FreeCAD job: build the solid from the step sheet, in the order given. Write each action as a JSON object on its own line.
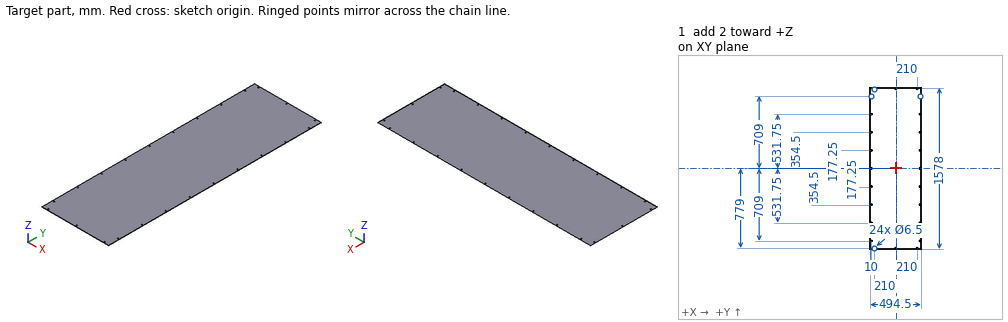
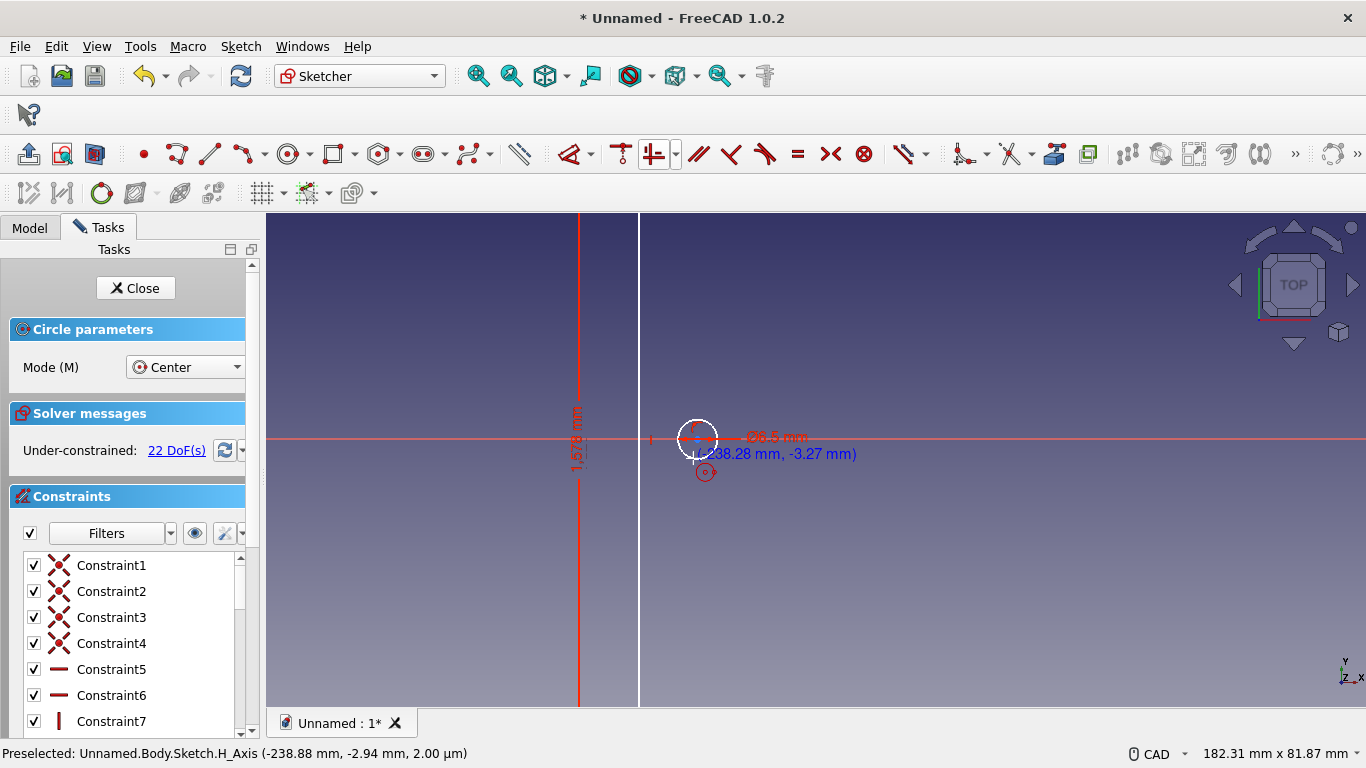
{"action": "scroll", "coordinate": [700, 461], "scroll_direction": "down", "scroll_amount": 17}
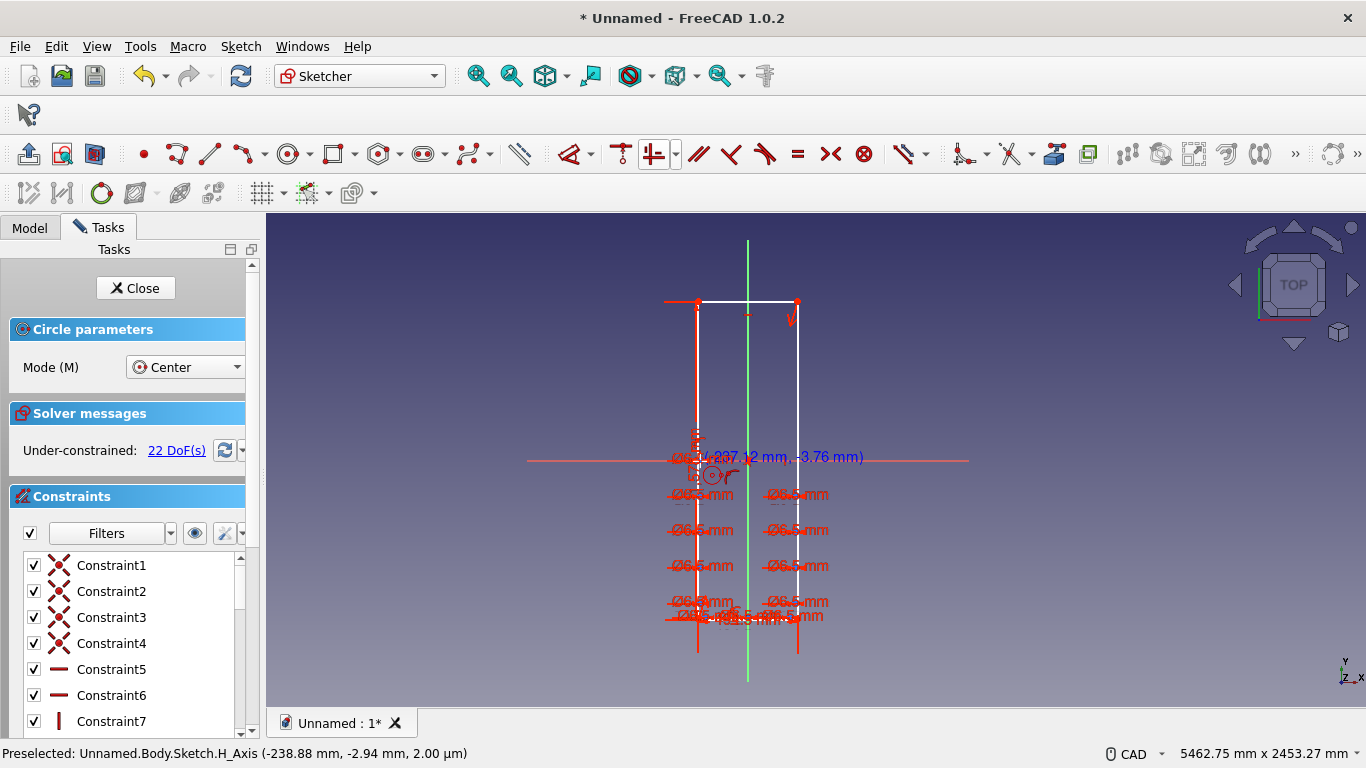
{"action": "scroll", "coordinate": [700, 425], "scroll_direction": "up", "scroll_amount": 18}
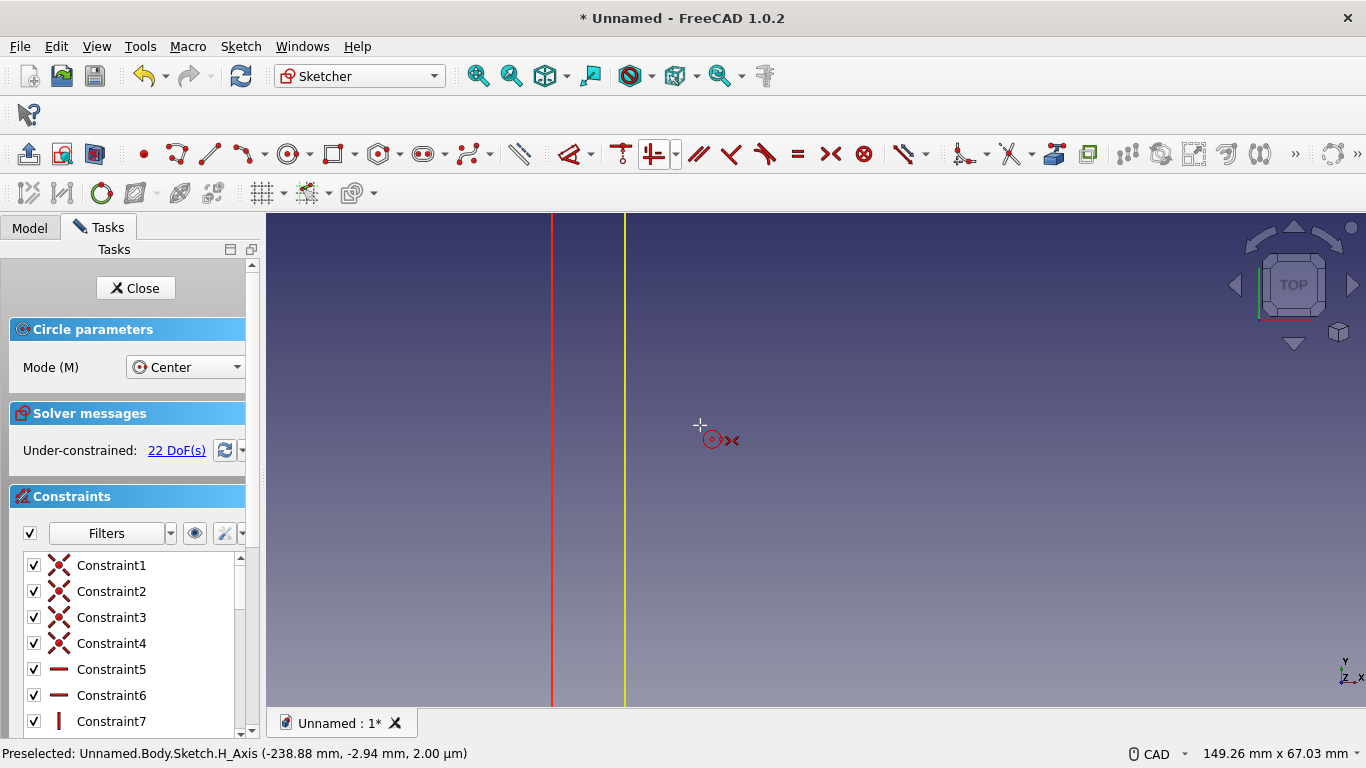
{"action": "scroll", "coordinate": [700, 425], "scroll_direction": "down", "scroll_amount": 18}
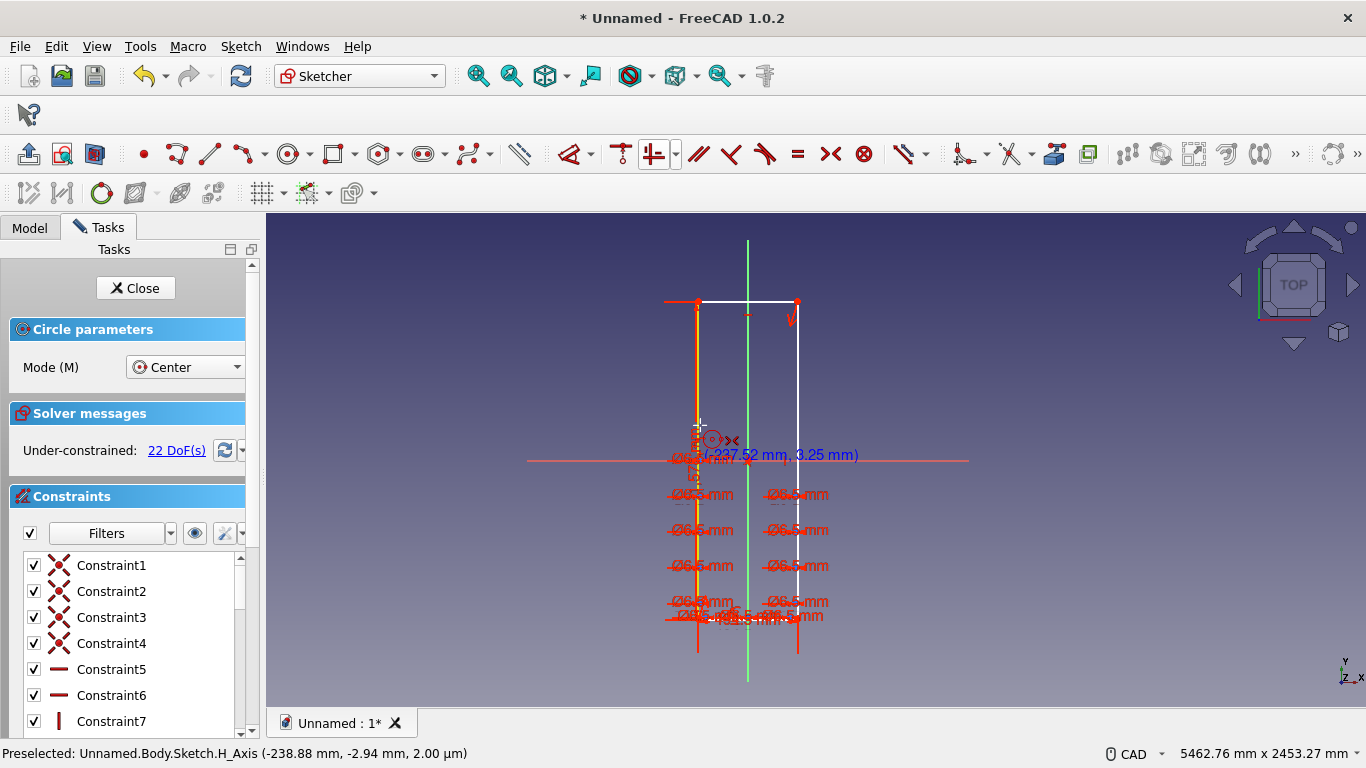
{"action": "scroll", "coordinate": [700, 425], "scroll_direction": "up", "scroll_amount": 11}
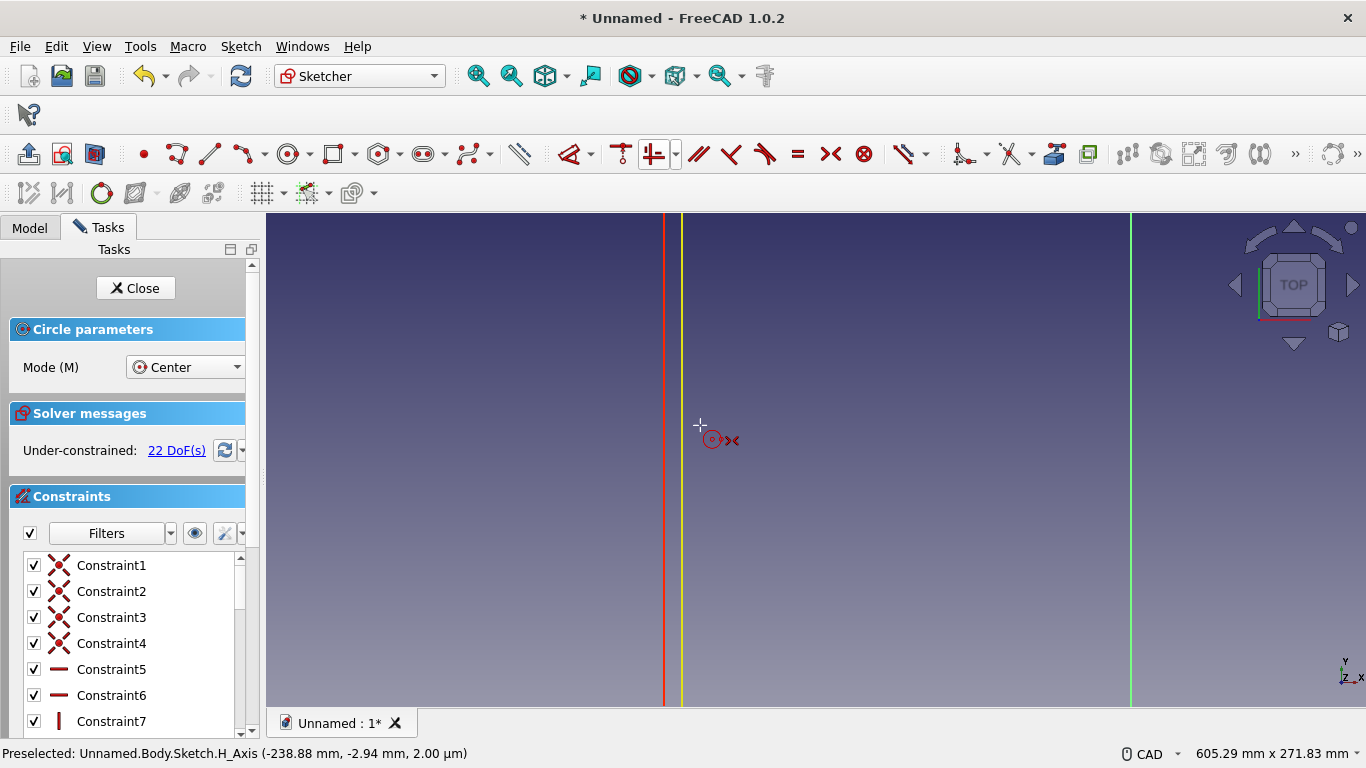
{"action": "left_click", "coordinate": [700, 422]}
{"action": "mouse_move", "coordinate": [704, 418]}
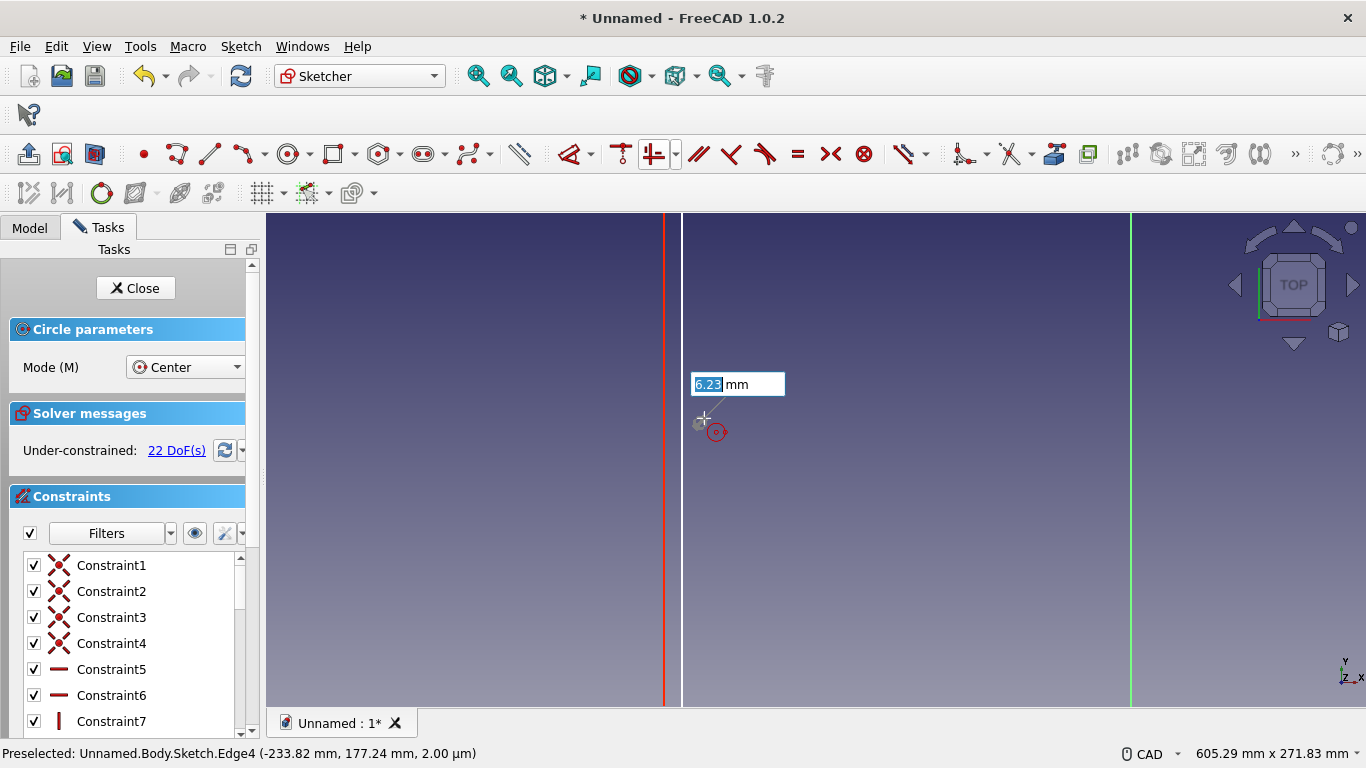
{"action": "type", "text": "6.5"}
{"action": "key", "text": "Return"}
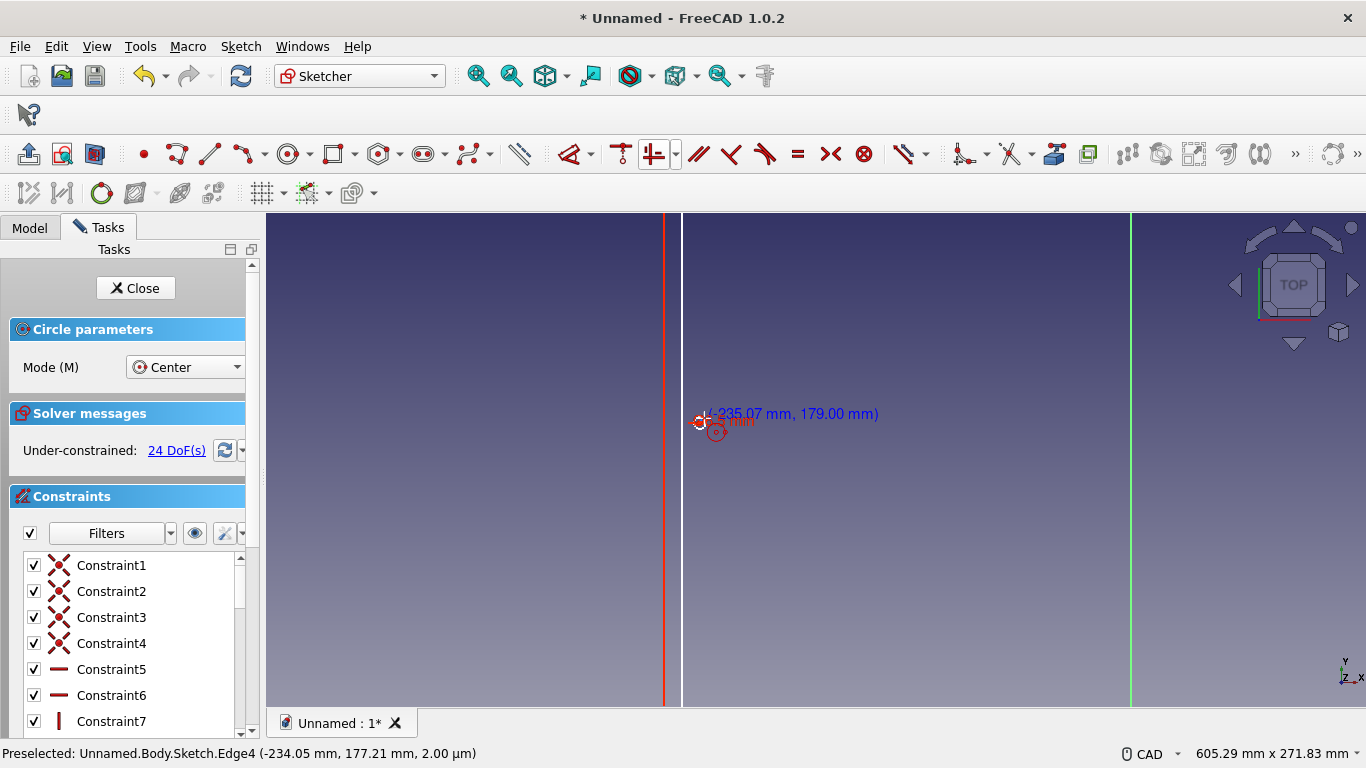
{"action": "scroll", "coordinate": [700, 425], "scroll_direction": "down", "scroll_amount": 11}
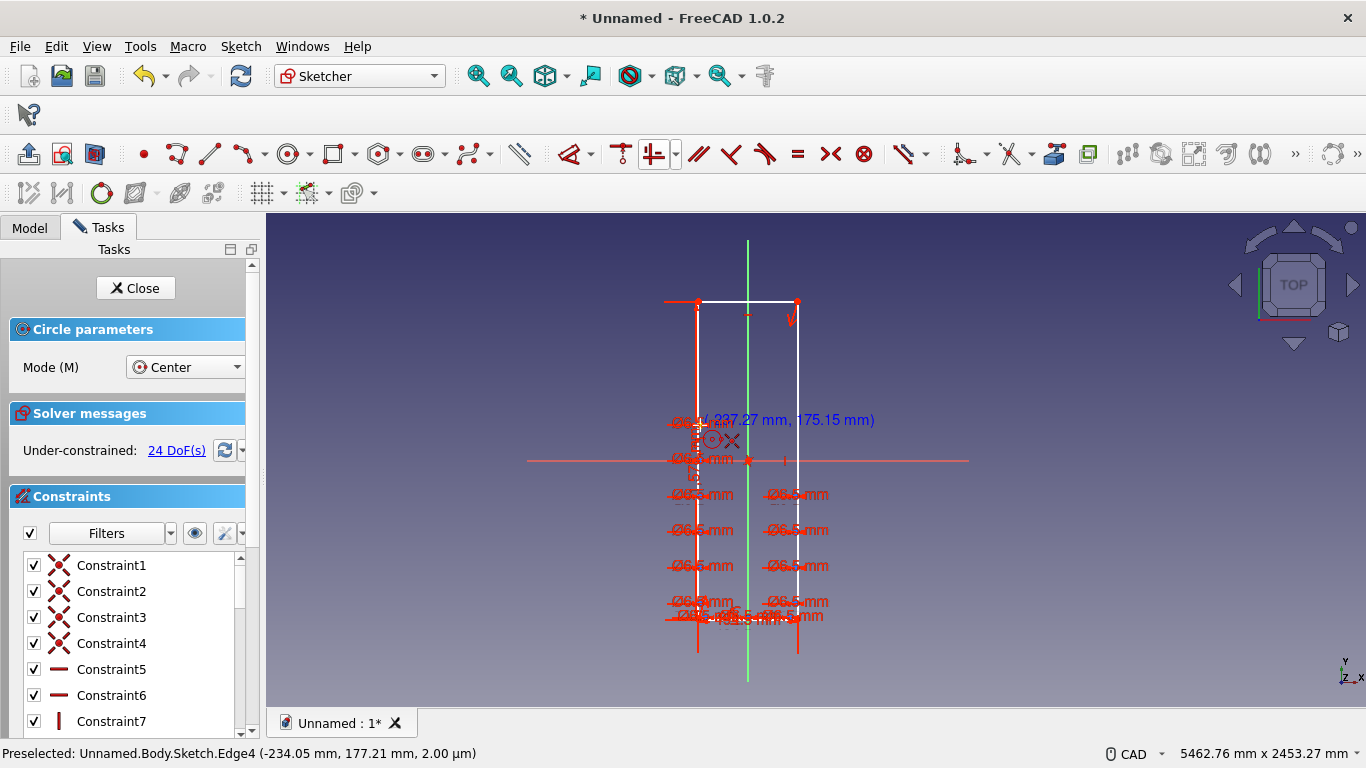
{"action": "scroll", "coordinate": [700, 389], "scroll_direction": "up", "scroll_amount": 18}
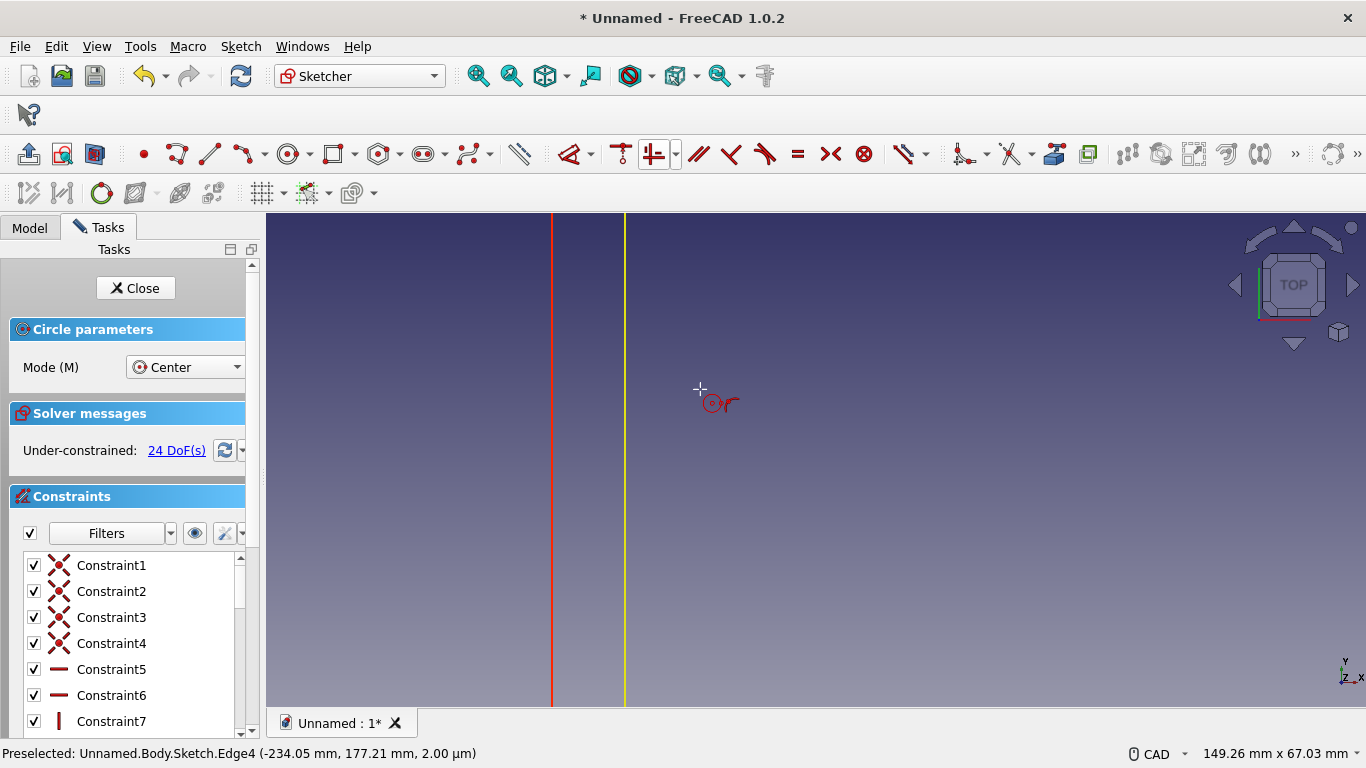
{"action": "scroll", "coordinate": [700, 389], "scroll_direction": "down", "scroll_amount": 18}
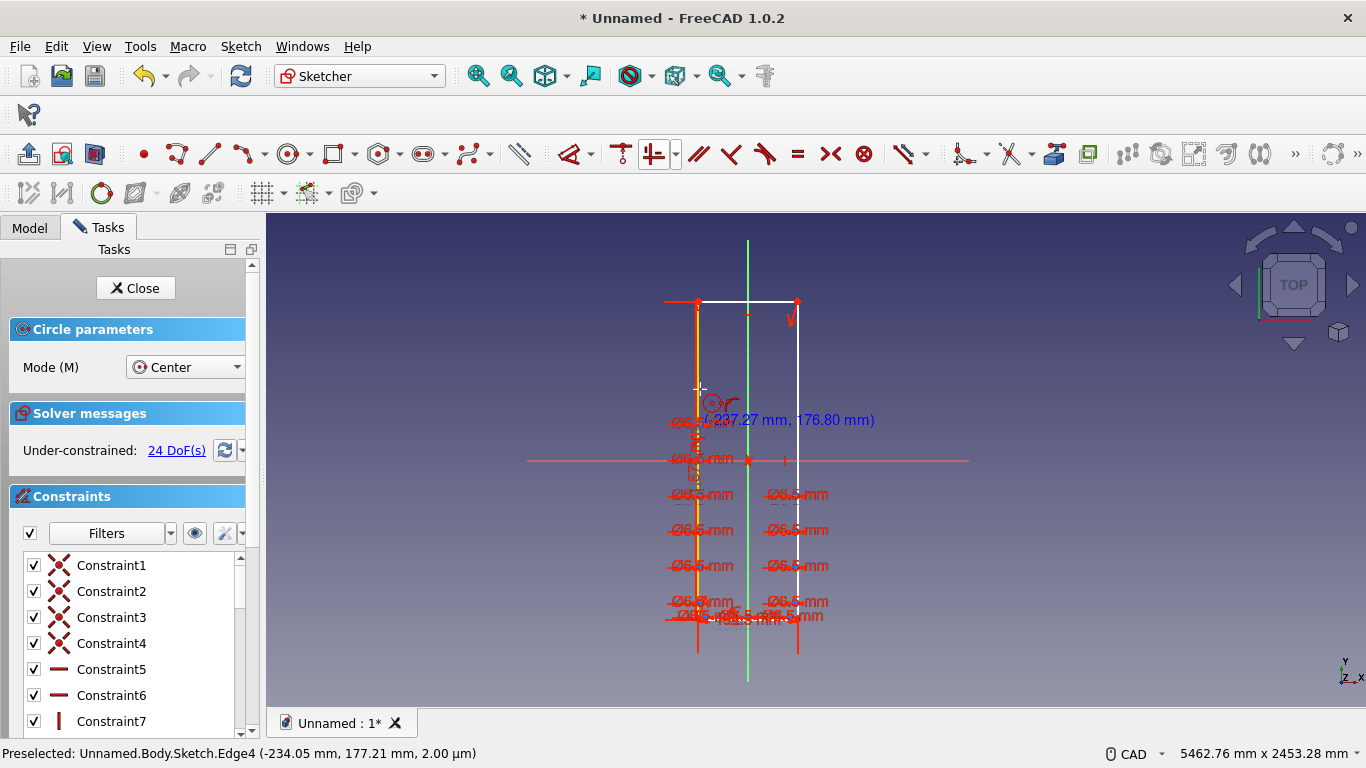
{"action": "scroll", "coordinate": [700, 389], "scroll_direction": "up", "scroll_amount": 11}